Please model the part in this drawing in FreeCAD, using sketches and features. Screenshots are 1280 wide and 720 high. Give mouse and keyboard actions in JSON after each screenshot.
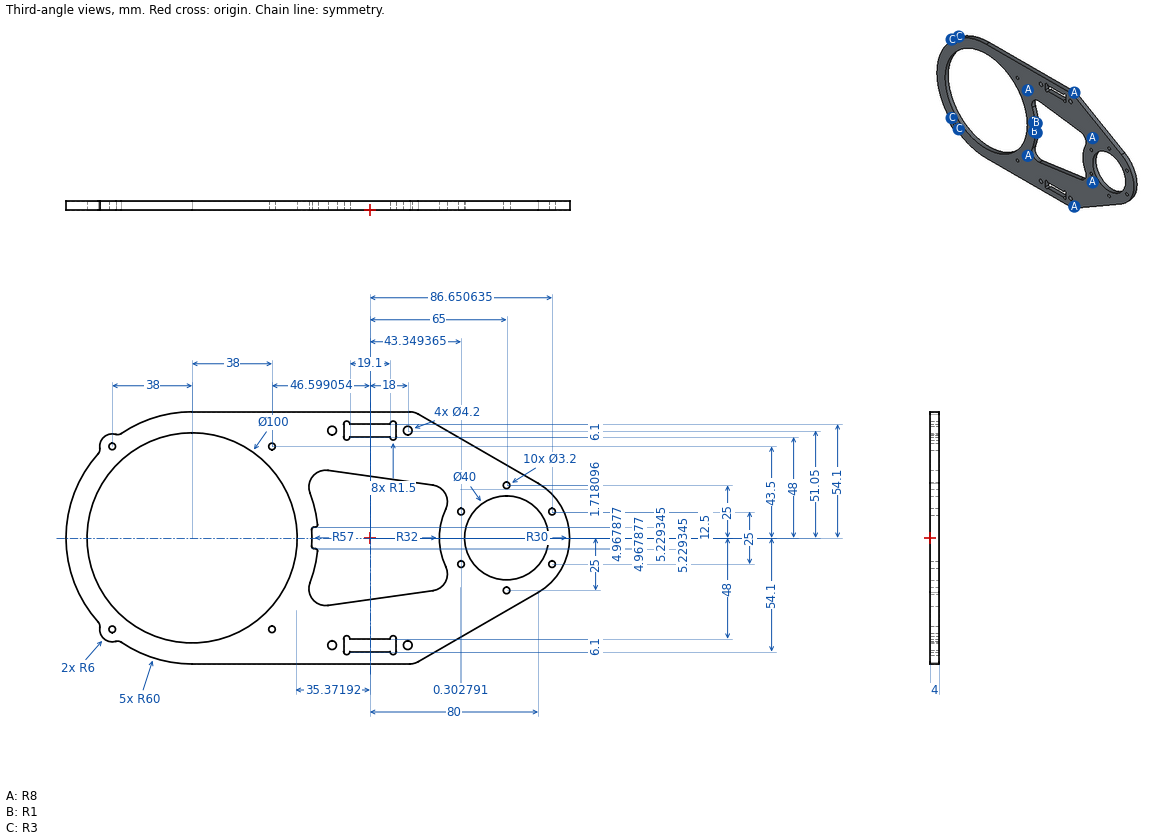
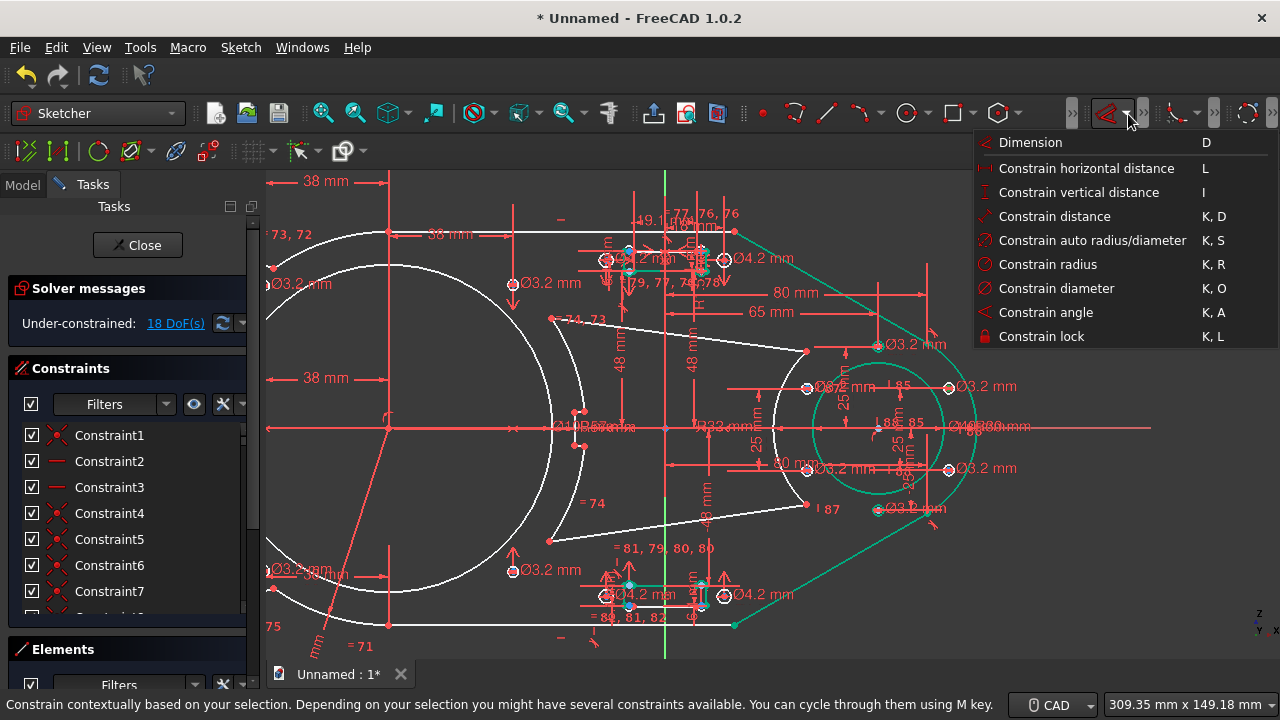
{"action": "left_click", "coordinate": [1126, 192]}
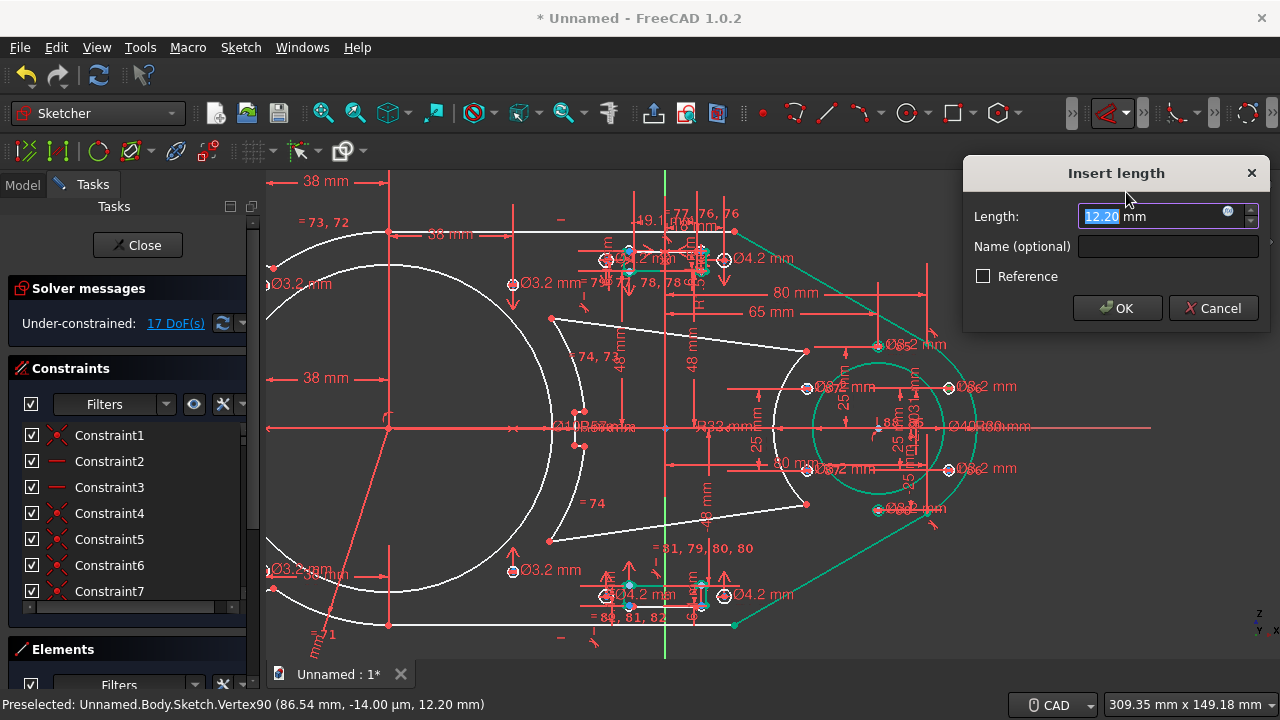
{"action": "type", "text": "12.5"}
{"action": "key", "text": "Return"}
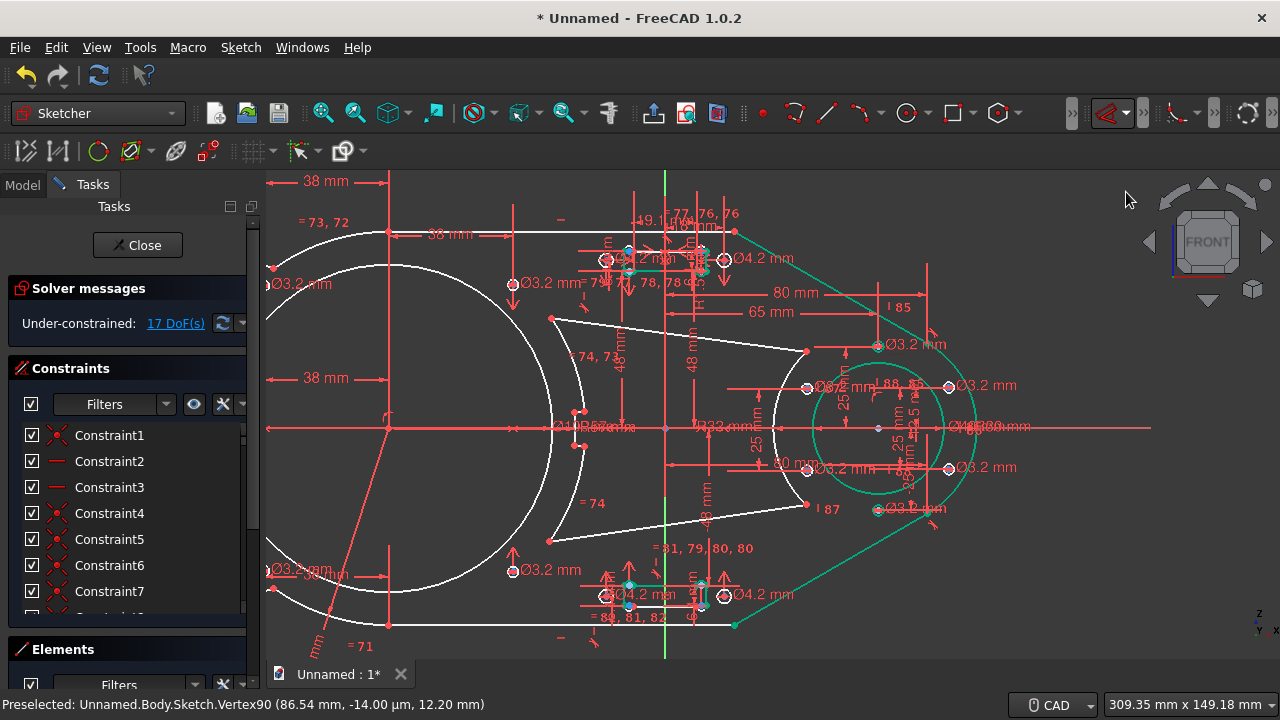
{"action": "left_click", "coordinate": [807, 389]}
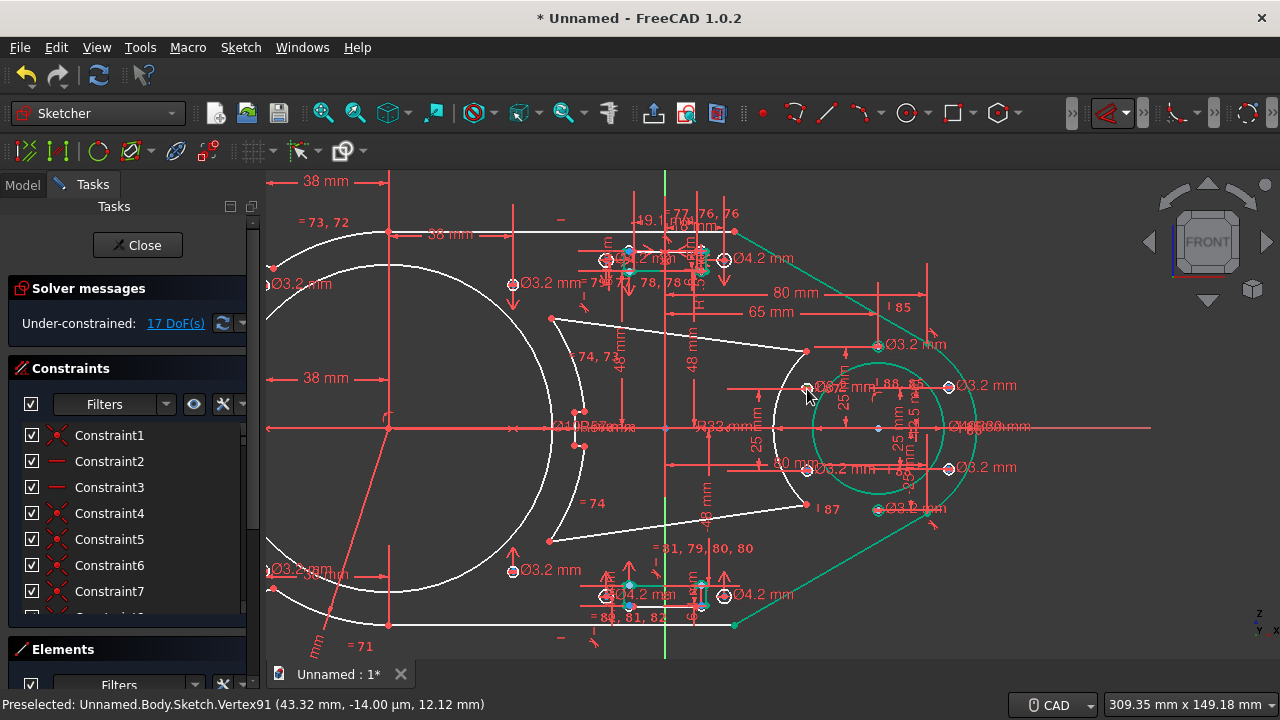
{"action": "key", "text": "i"}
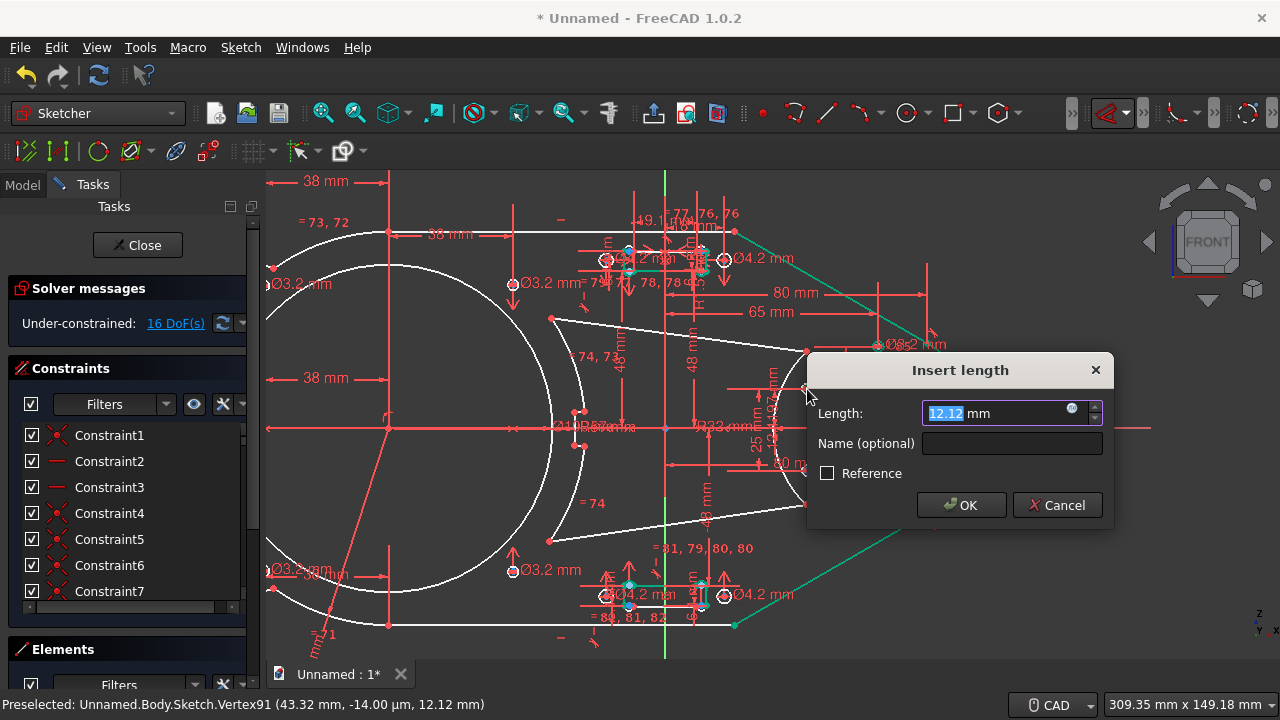
{"action": "type", "text": "12.5"}
{"action": "key", "text": "Return"}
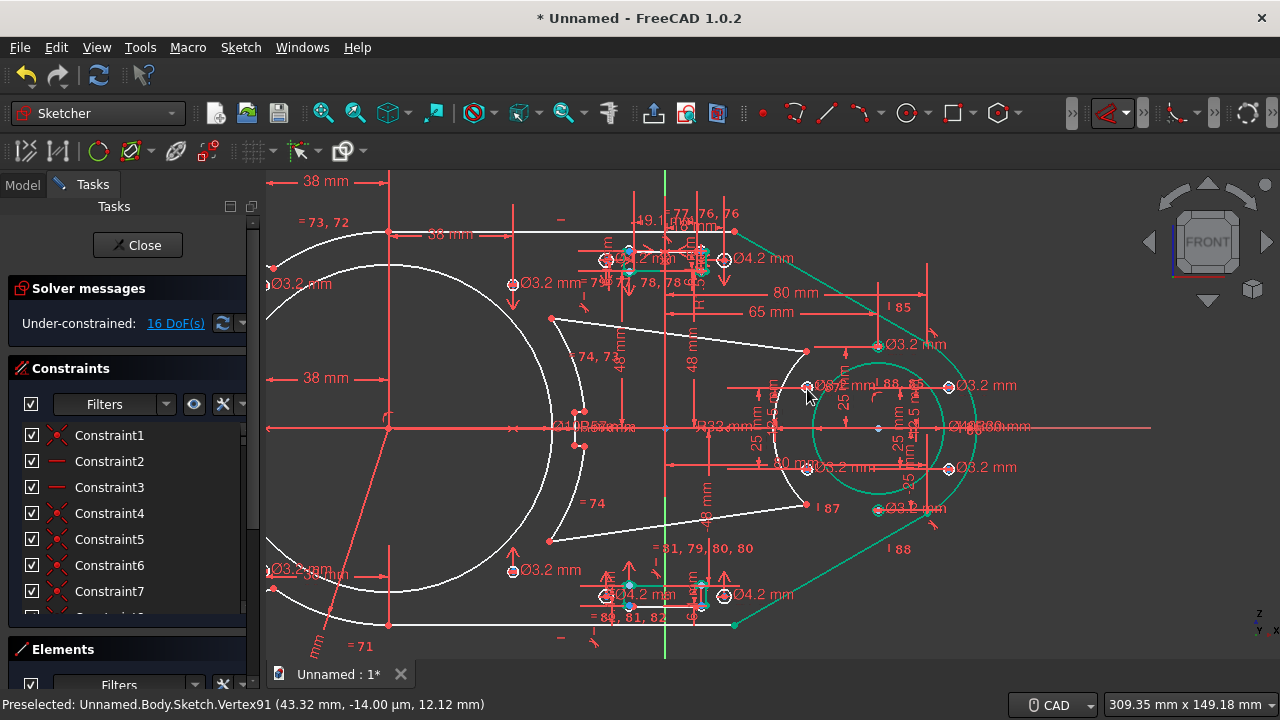
{"action": "left_click", "coordinate": [513, 285]}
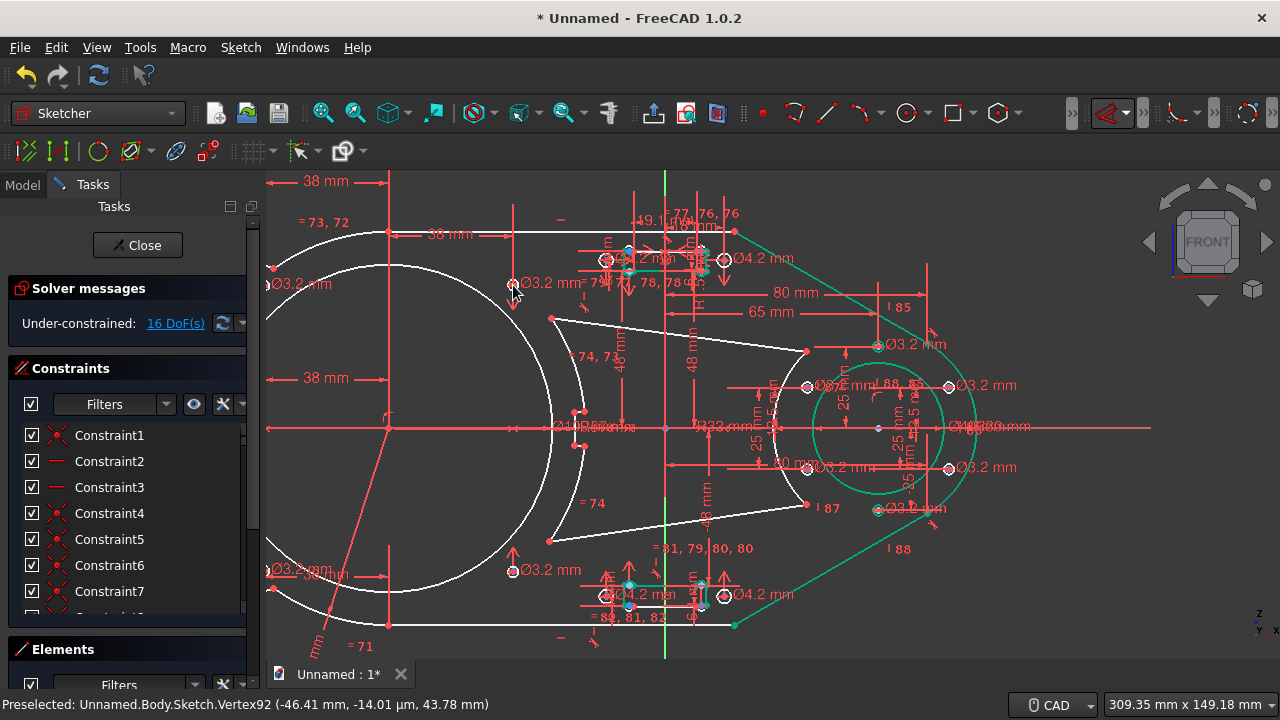
{"action": "left_click", "coordinate": [1128, 114]}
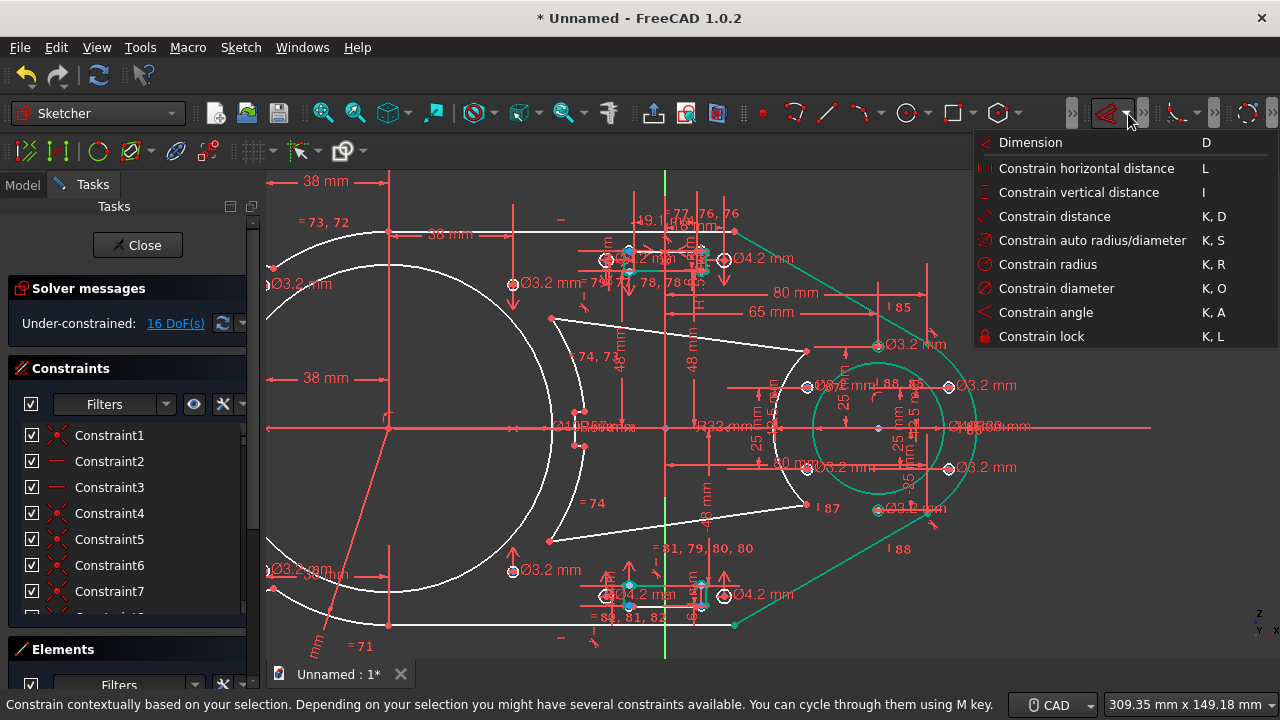
{"action": "left_click", "coordinate": [1126, 192]}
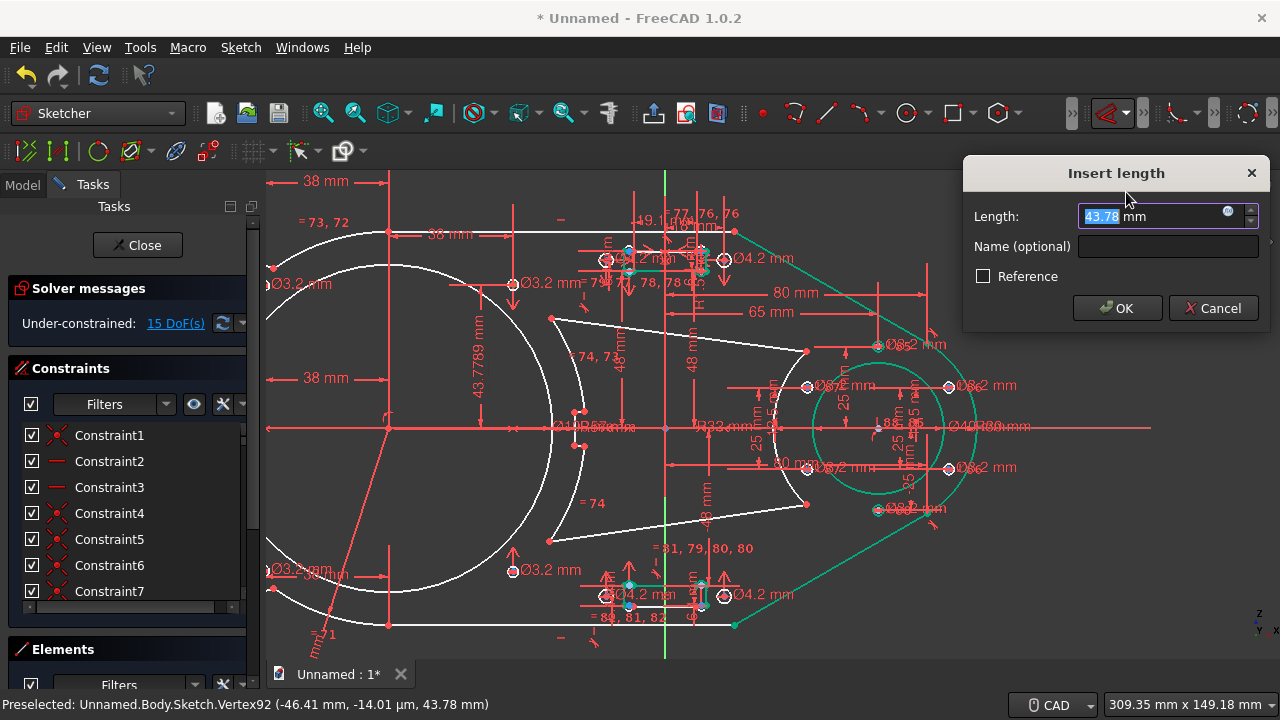
{"action": "type", "text": "43.5"}
{"action": "key", "text": "Return"}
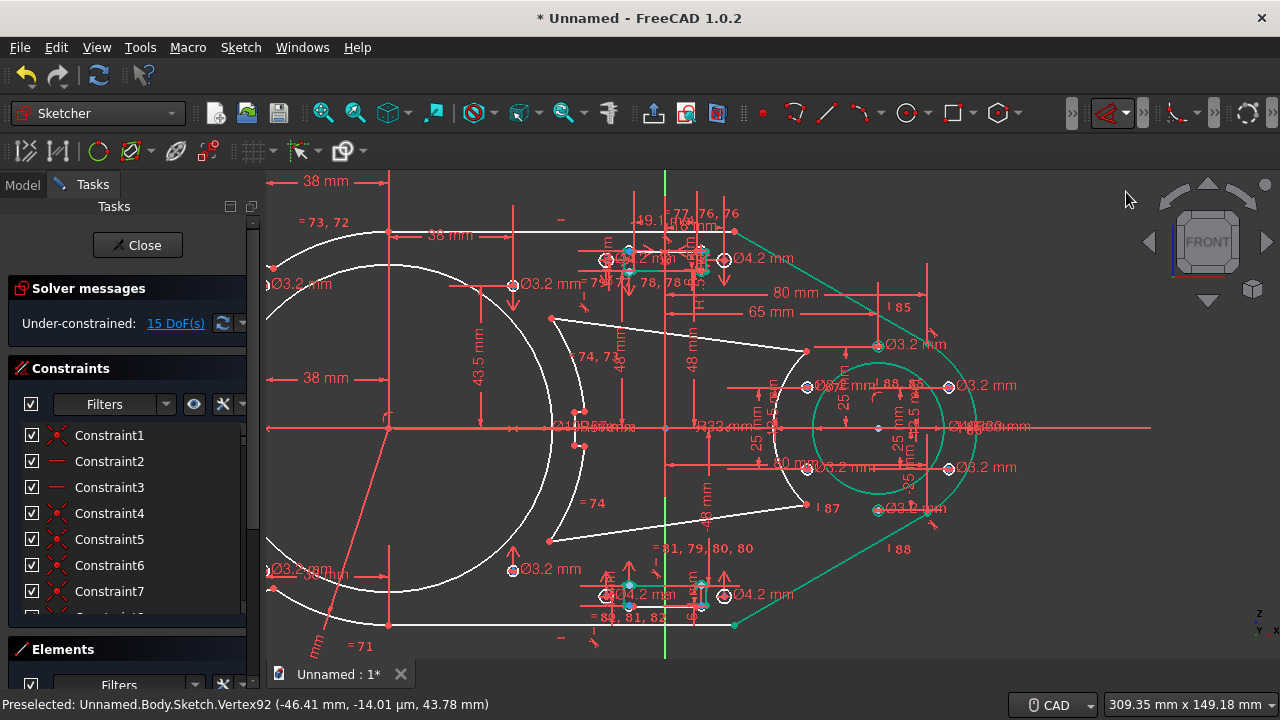
{"action": "scroll", "coordinate": [950, 386], "scroll_direction": "down", "scroll_amount": 2}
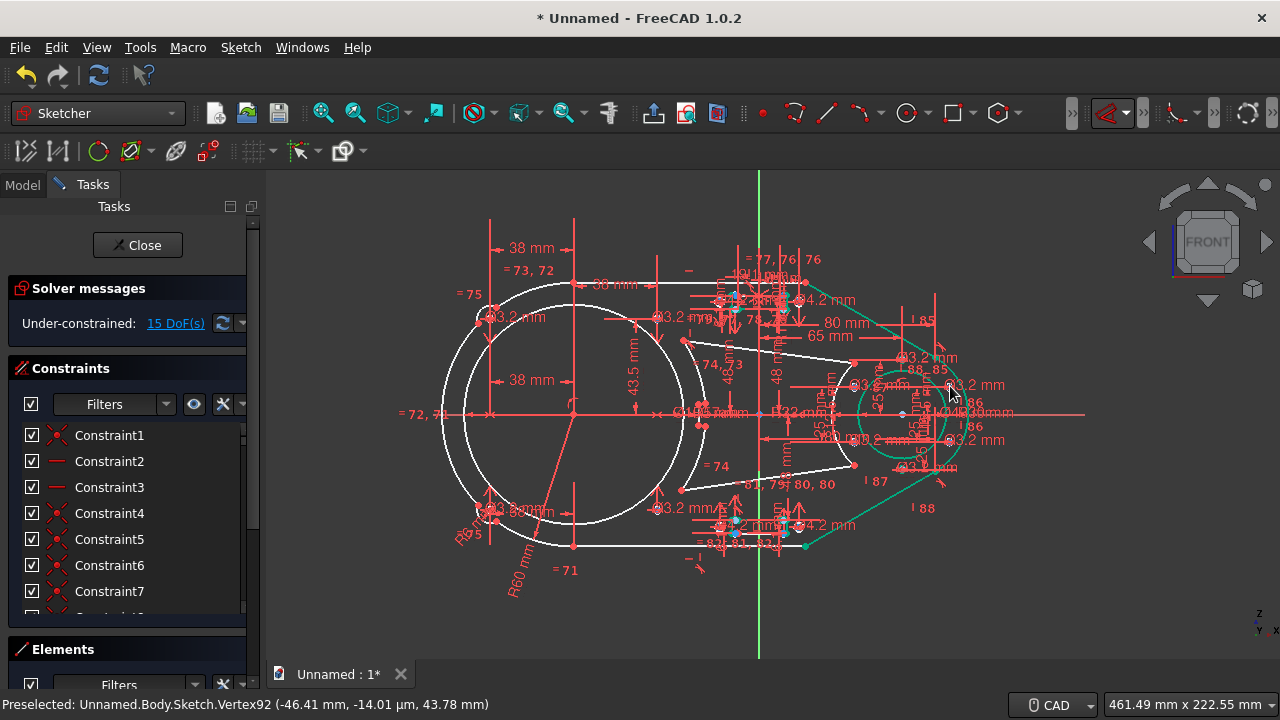
{"action": "left_click", "coordinate": [490, 319]}